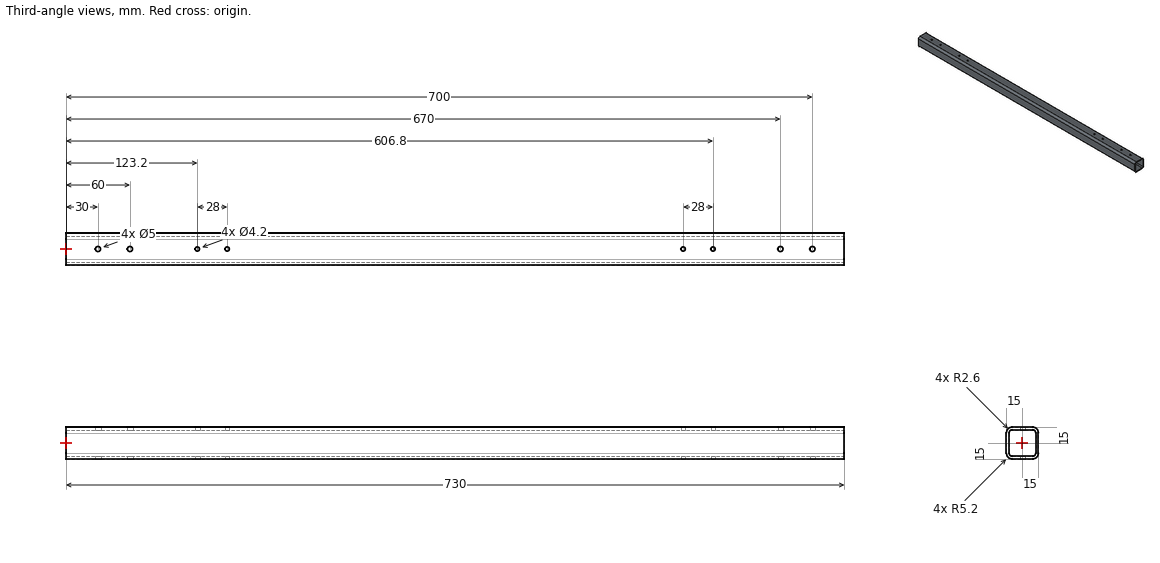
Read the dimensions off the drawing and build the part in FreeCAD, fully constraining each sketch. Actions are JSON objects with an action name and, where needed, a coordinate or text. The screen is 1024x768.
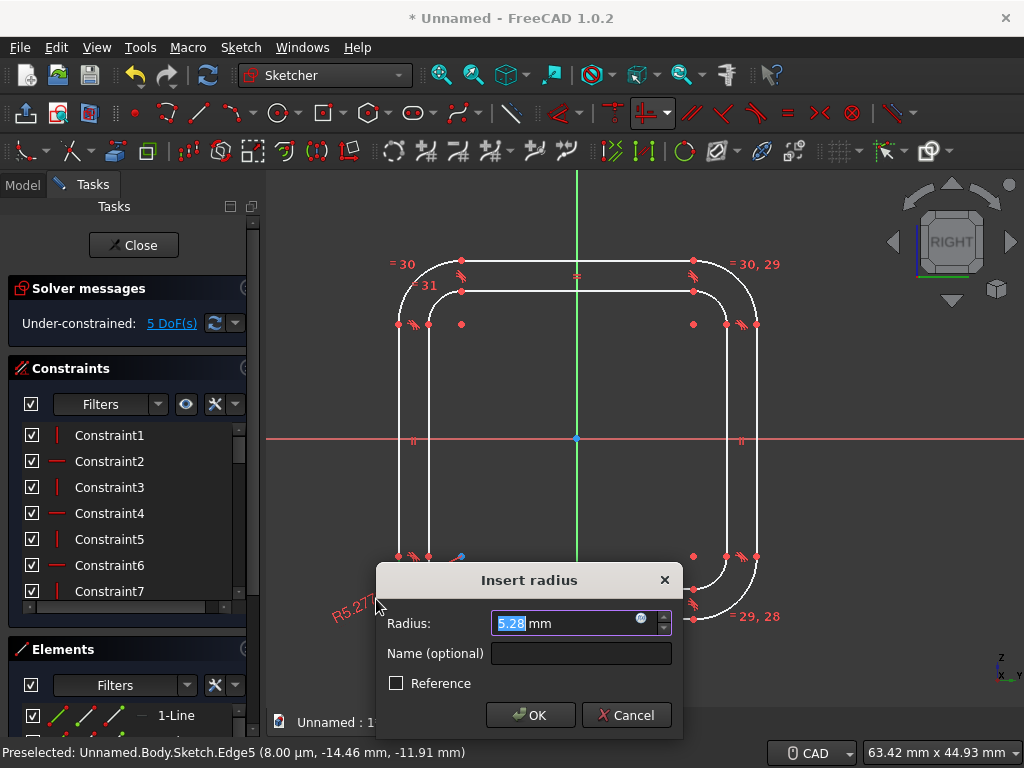
{"action": "type", "text": "5.2"}
{"action": "key", "text": "Return"}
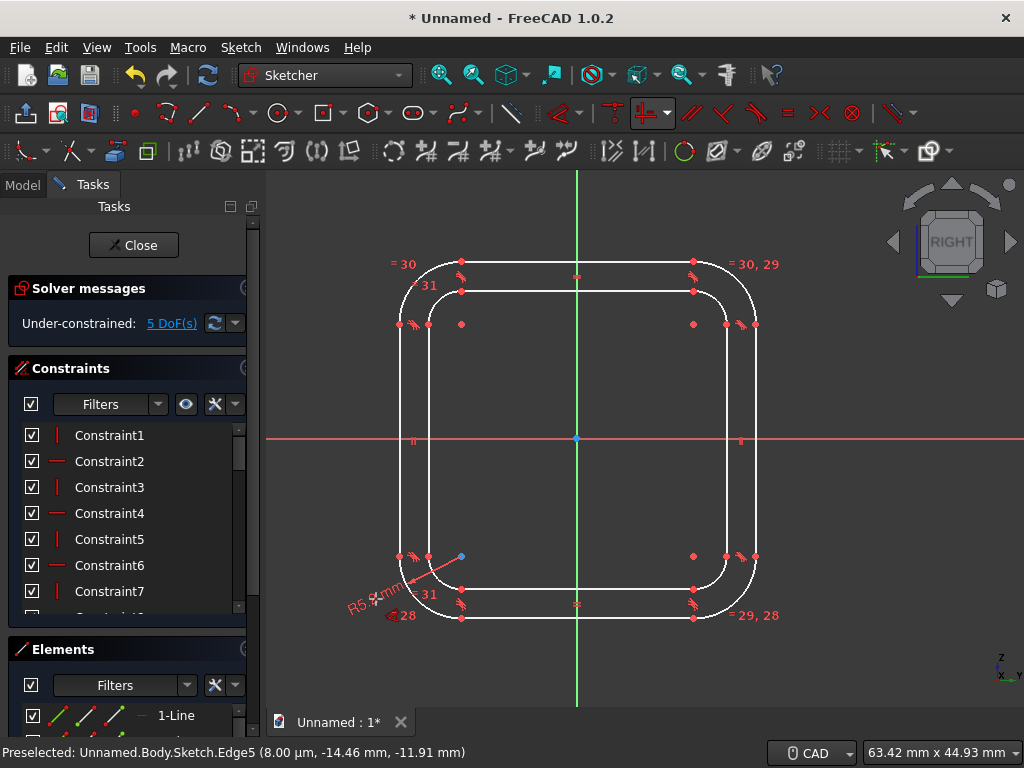
{"action": "scroll", "coordinate": [447, 295], "scroll_direction": "up", "scroll_amount": 2}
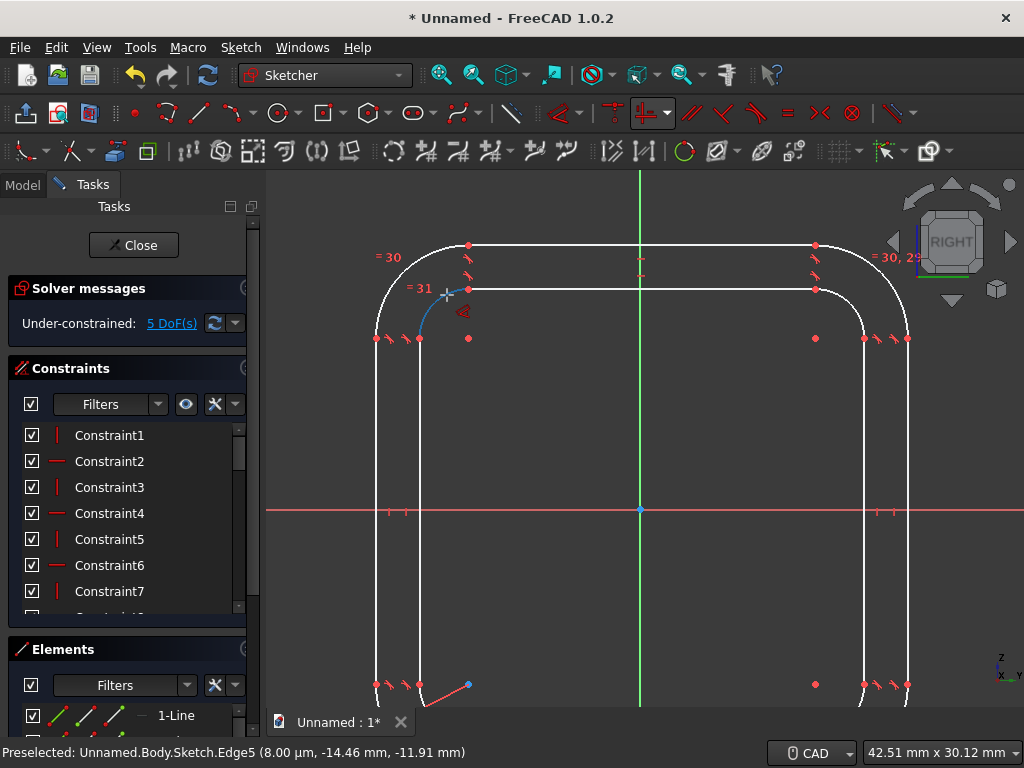
{"action": "left_click", "coordinate": [446, 294]}
{"action": "left_click", "coordinate": [510, 267]}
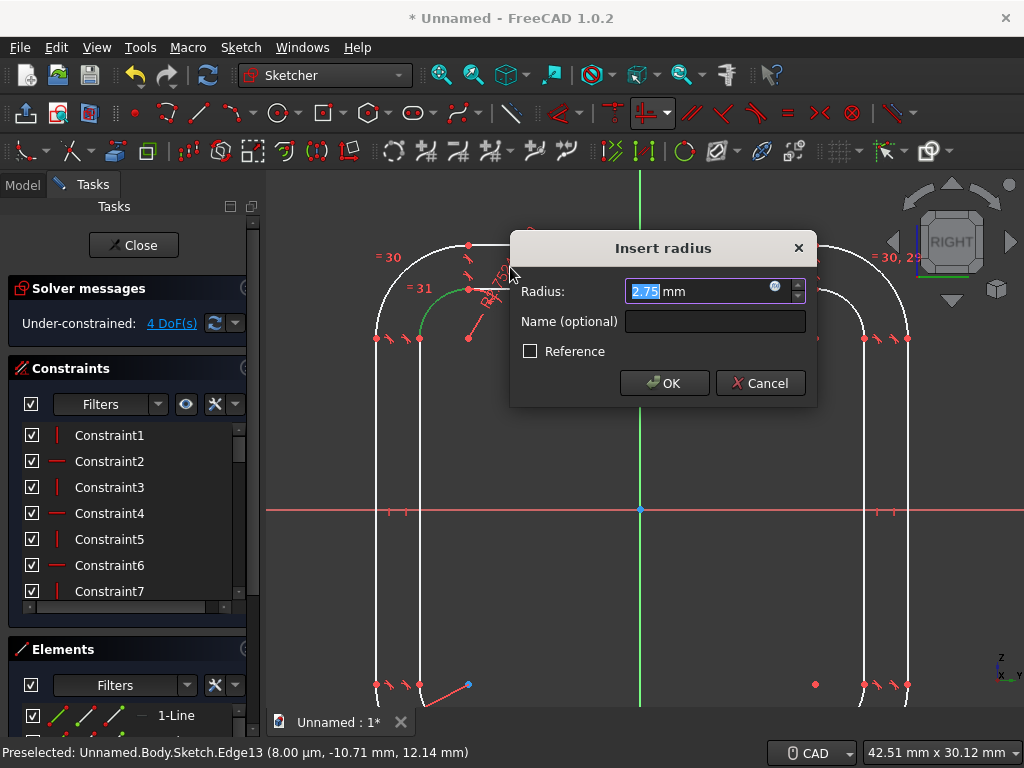
{"action": "type", "text": "2.6"}
{"action": "key", "text": "Return"}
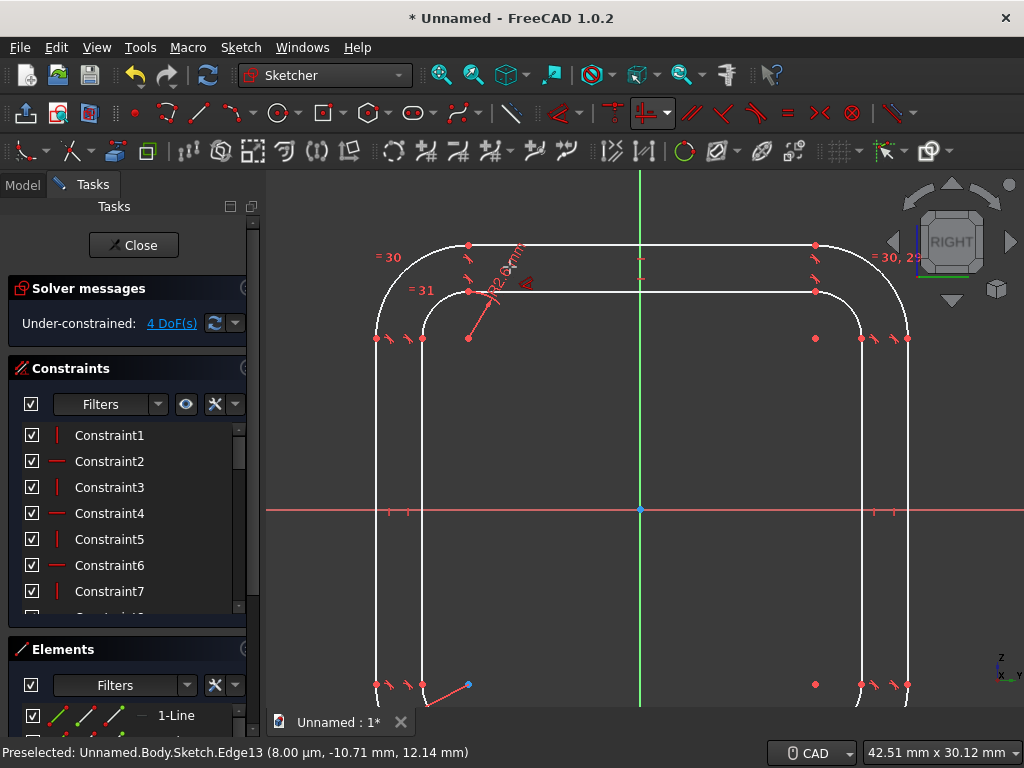
{"action": "left_click", "coordinate": [376, 338]}
{"action": "left_click", "coordinate": [416, 304]}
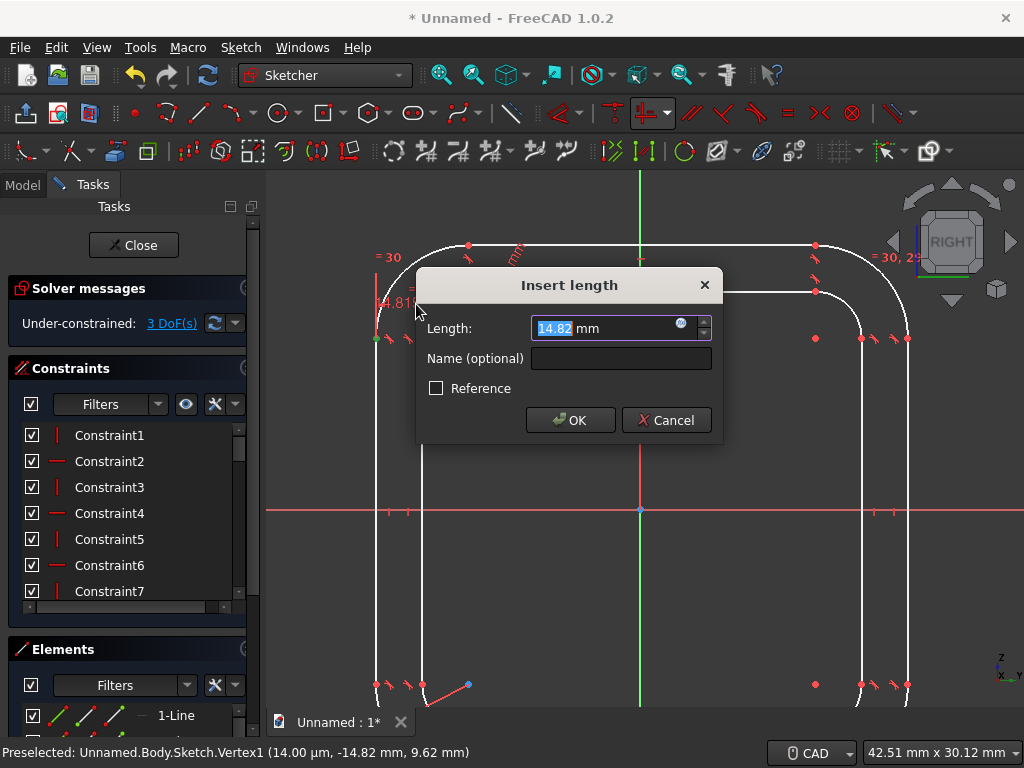
{"action": "type", "text": "15"}
{"action": "key", "text": "Return"}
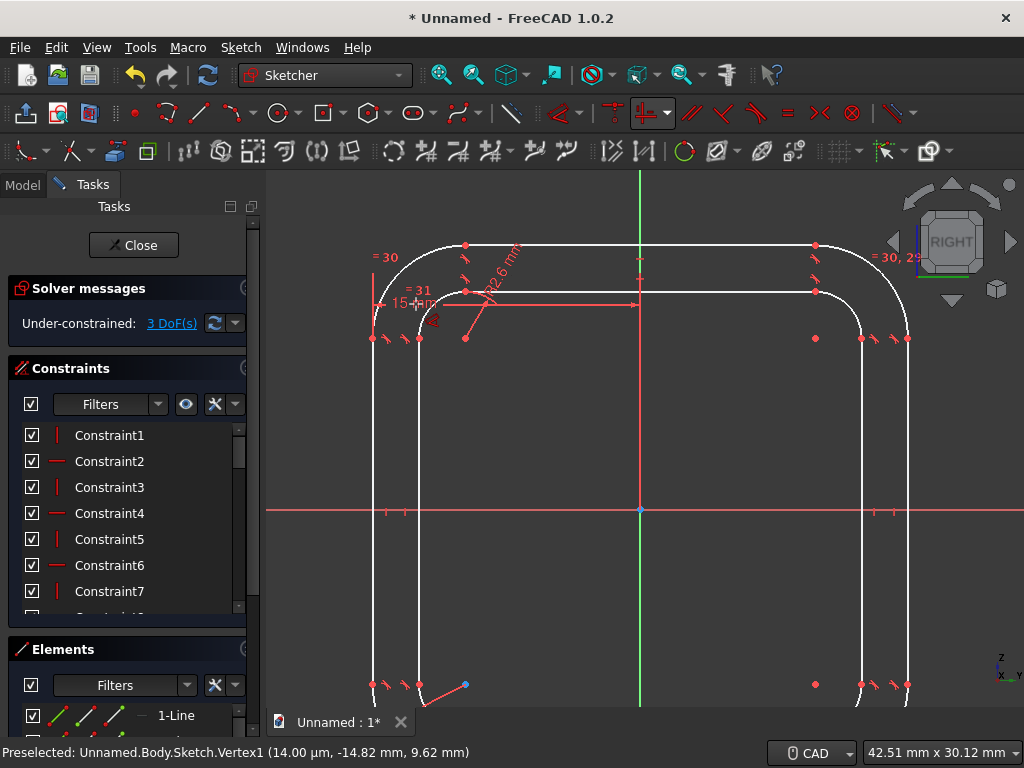
{"action": "scroll", "coordinate": [447, 294], "scroll_direction": "down", "scroll_amount": 2}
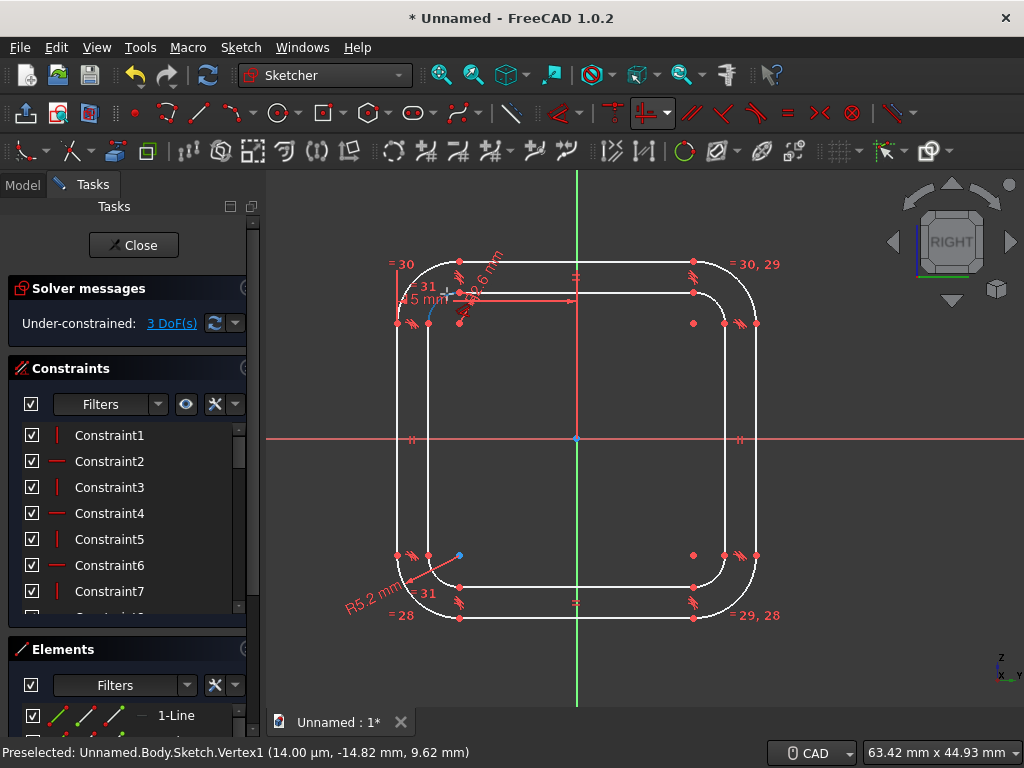
{"action": "left_click", "coordinate": [459, 618]}
{"action": "left_click", "coordinate": [611, 528]}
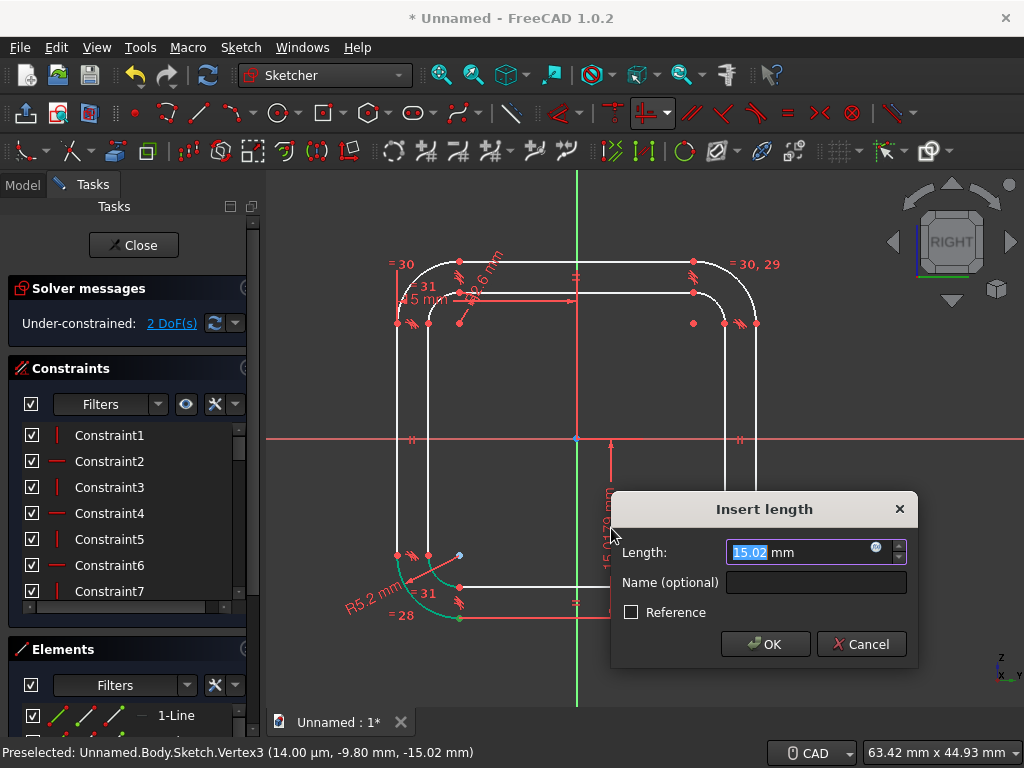
{"action": "type", "text": "15"}
{"action": "key", "text": "Return"}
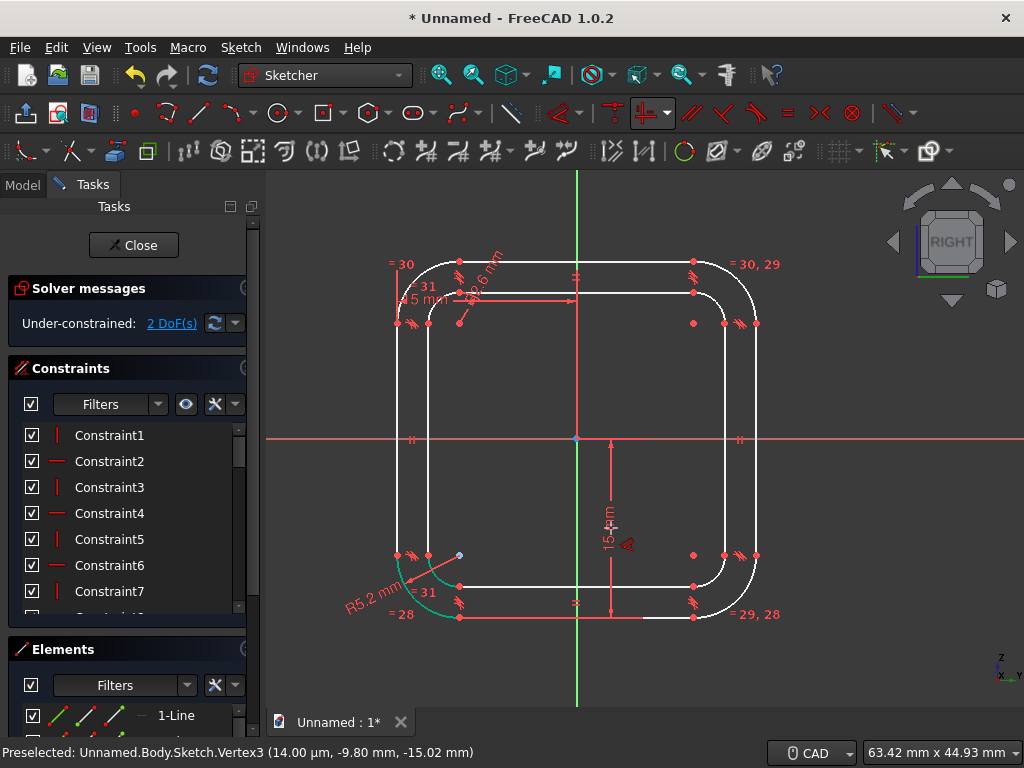
{"action": "left_click", "coordinate": [756, 556]}
{"action": "left_click", "coordinate": [729, 590]}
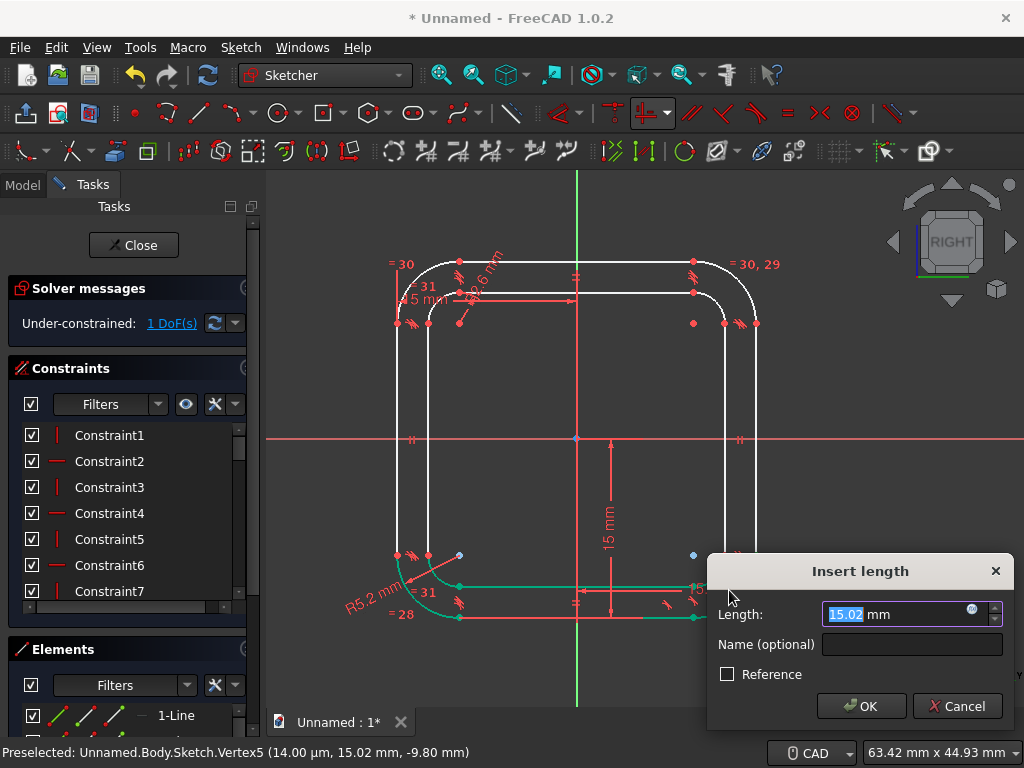
{"action": "type", "text": "15"}
{"action": "key", "text": "Return"}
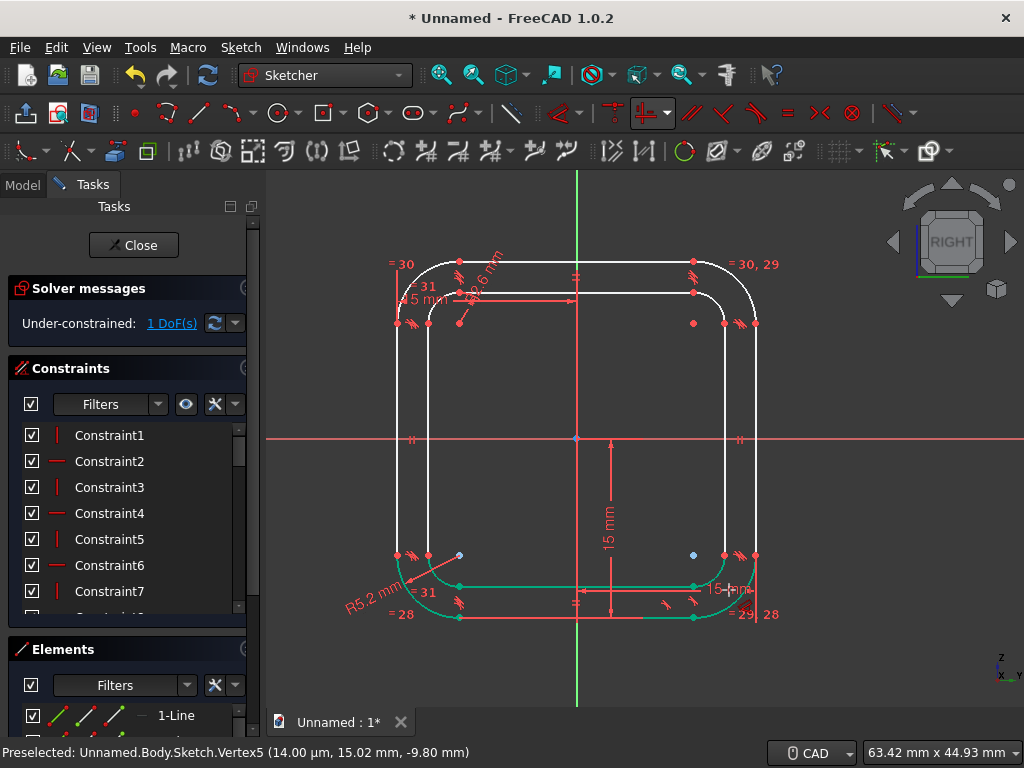
{"action": "left_click", "coordinate": [694, 262]}
{"action": "left_click", "coordinate": [543, 350]}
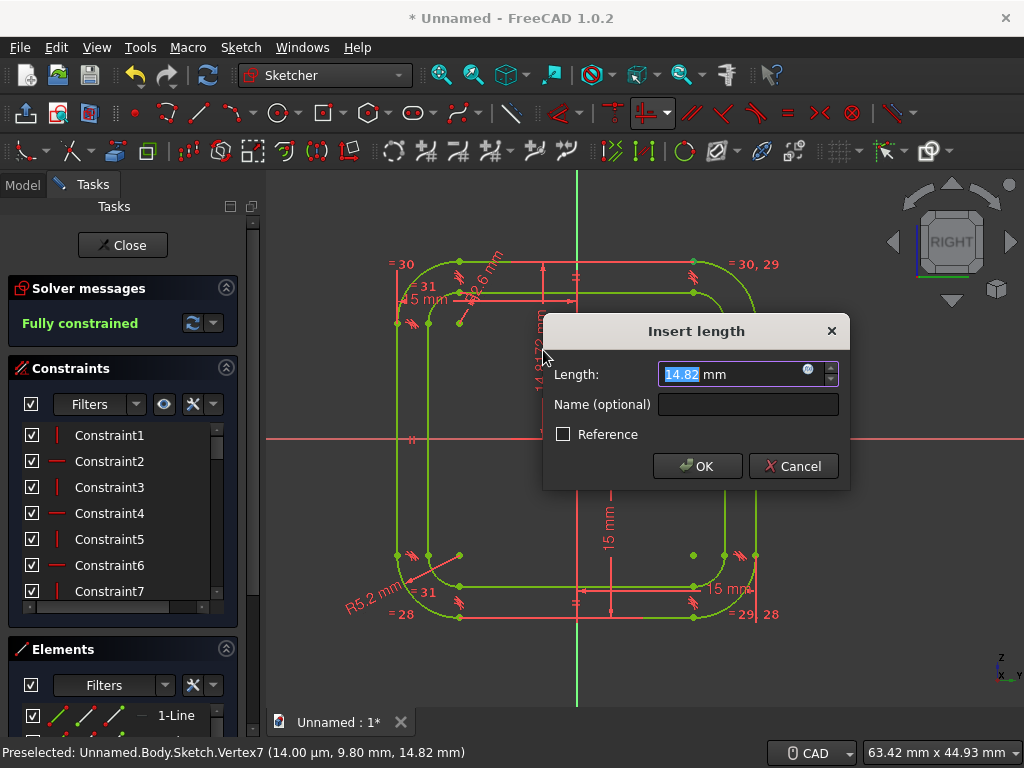
{"action": "type", "text": "15"}
{"action": "key", "text": "Return"}
{"action": "key", "text": "Escape"}